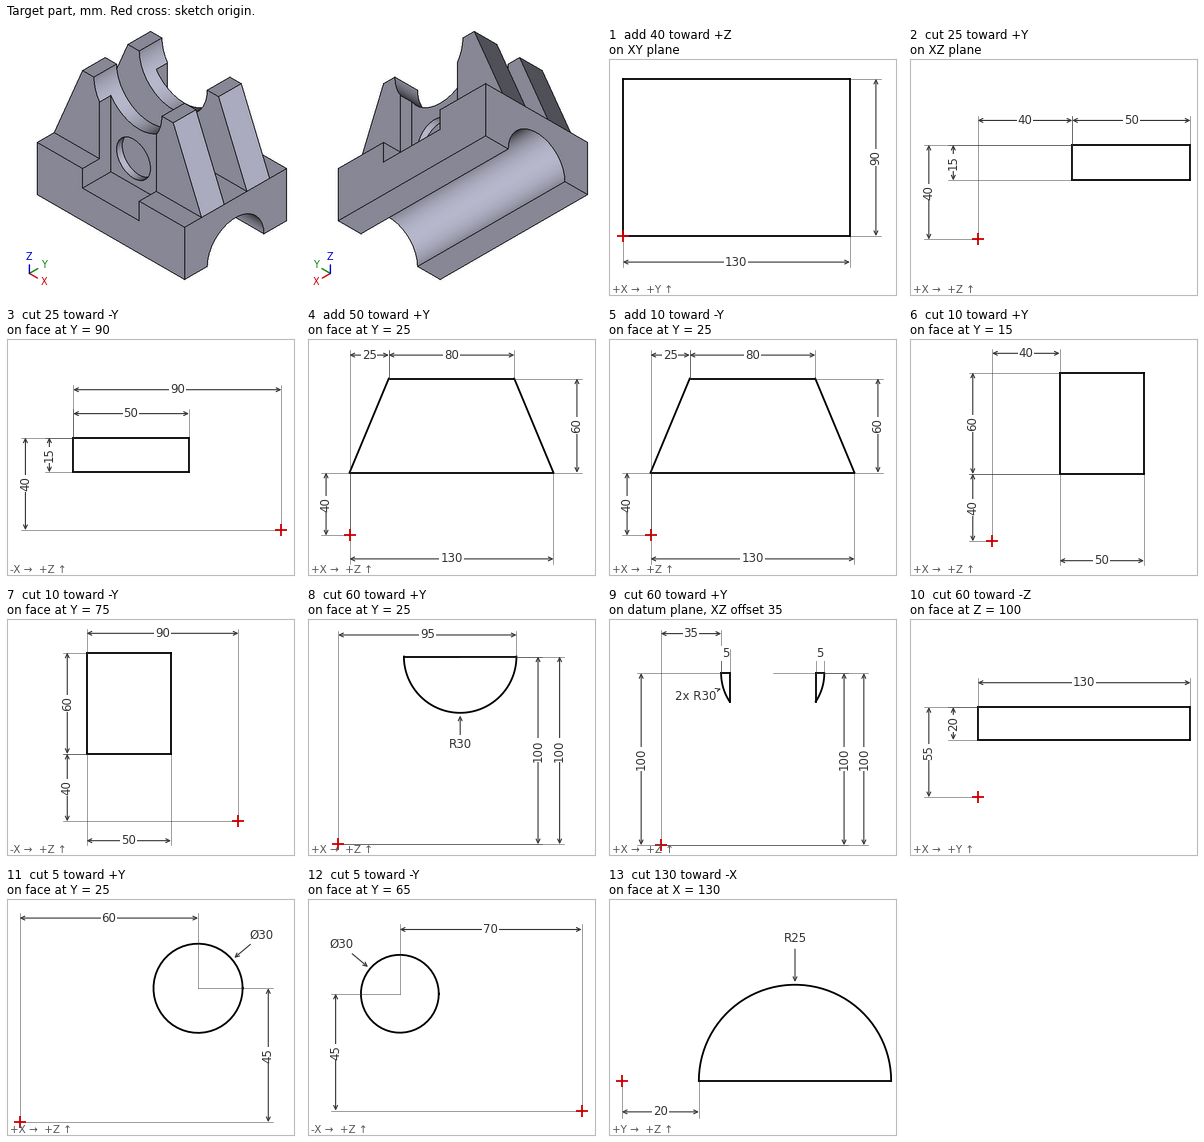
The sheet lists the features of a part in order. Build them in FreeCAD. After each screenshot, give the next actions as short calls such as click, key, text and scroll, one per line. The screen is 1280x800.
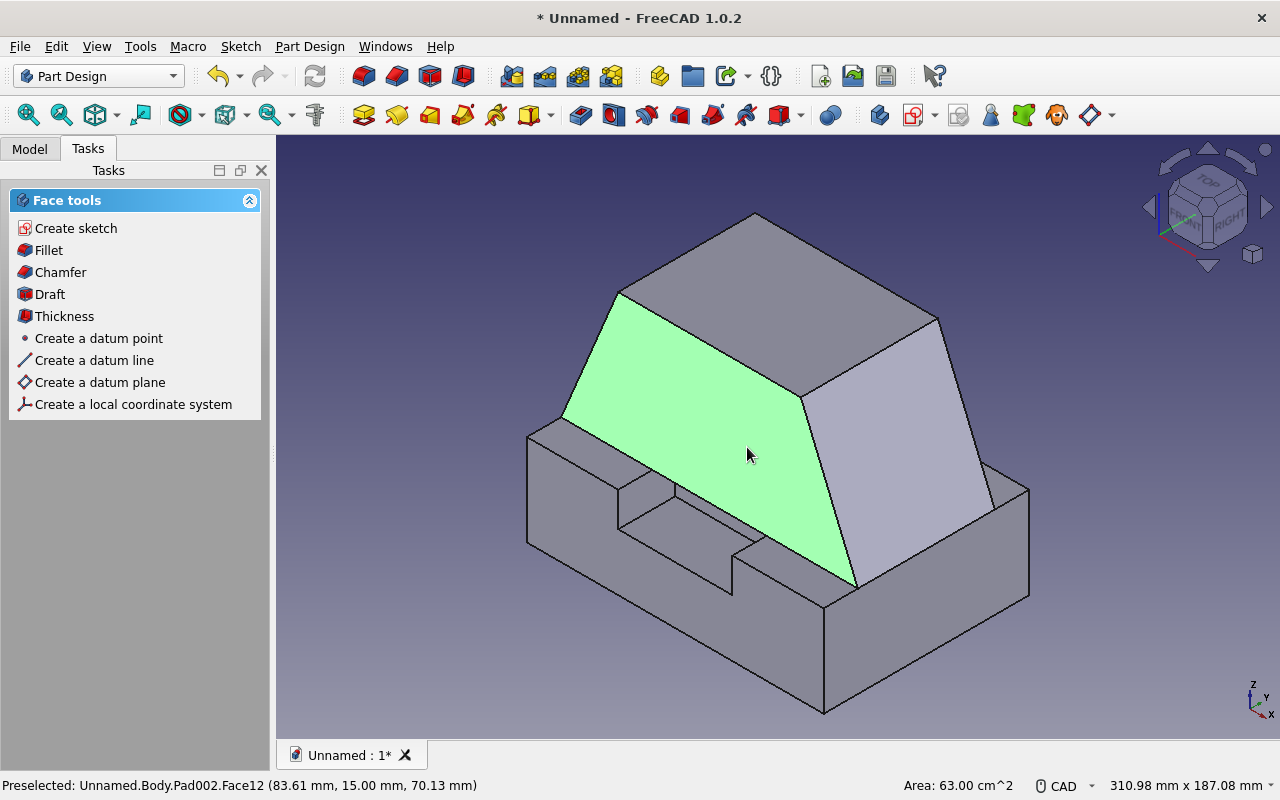
click(912, 116)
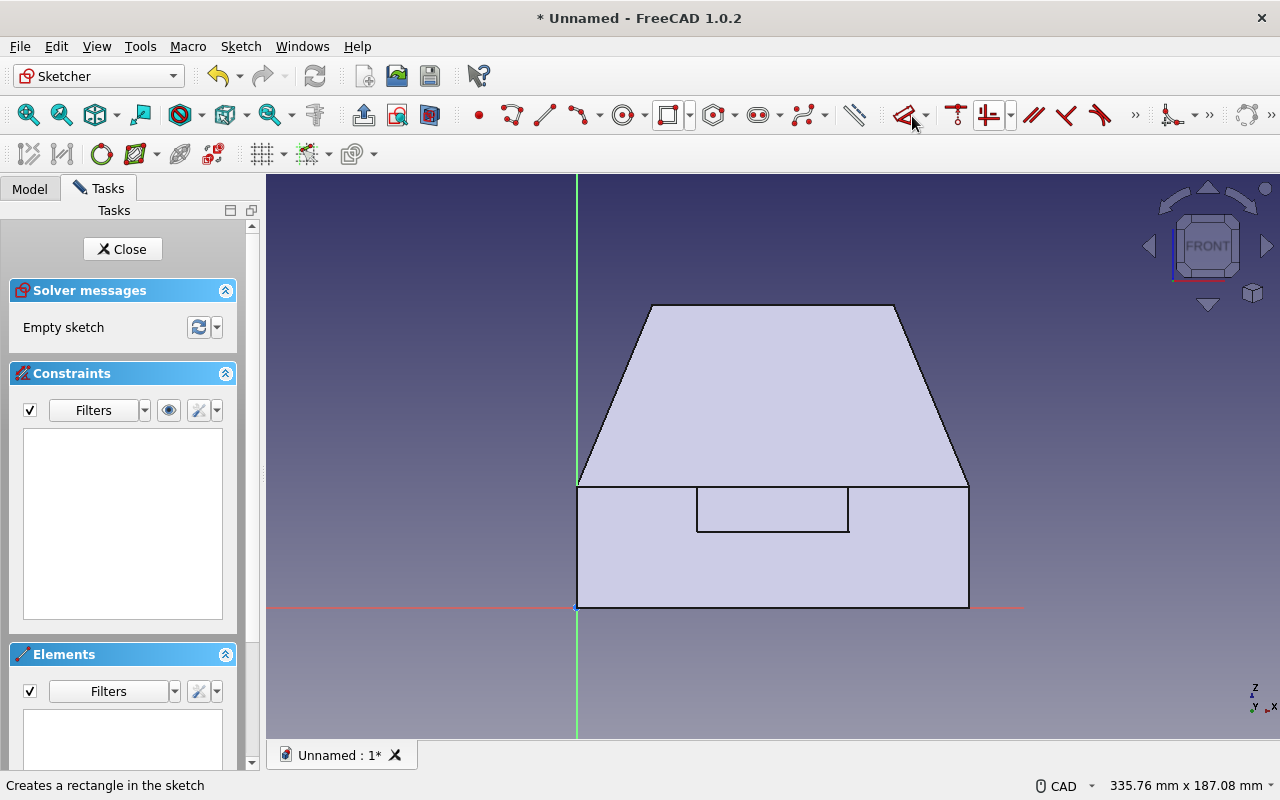
key(q)
key(s)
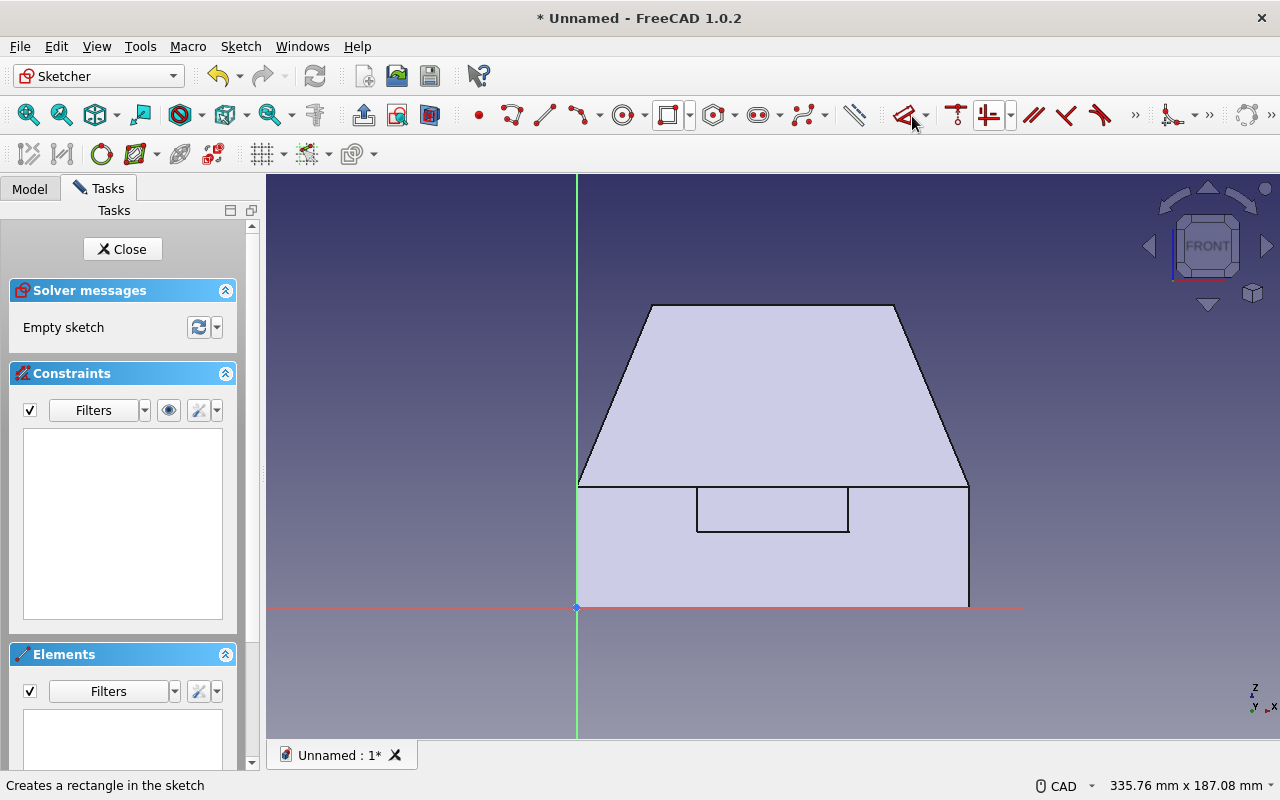
key(g)
key(r)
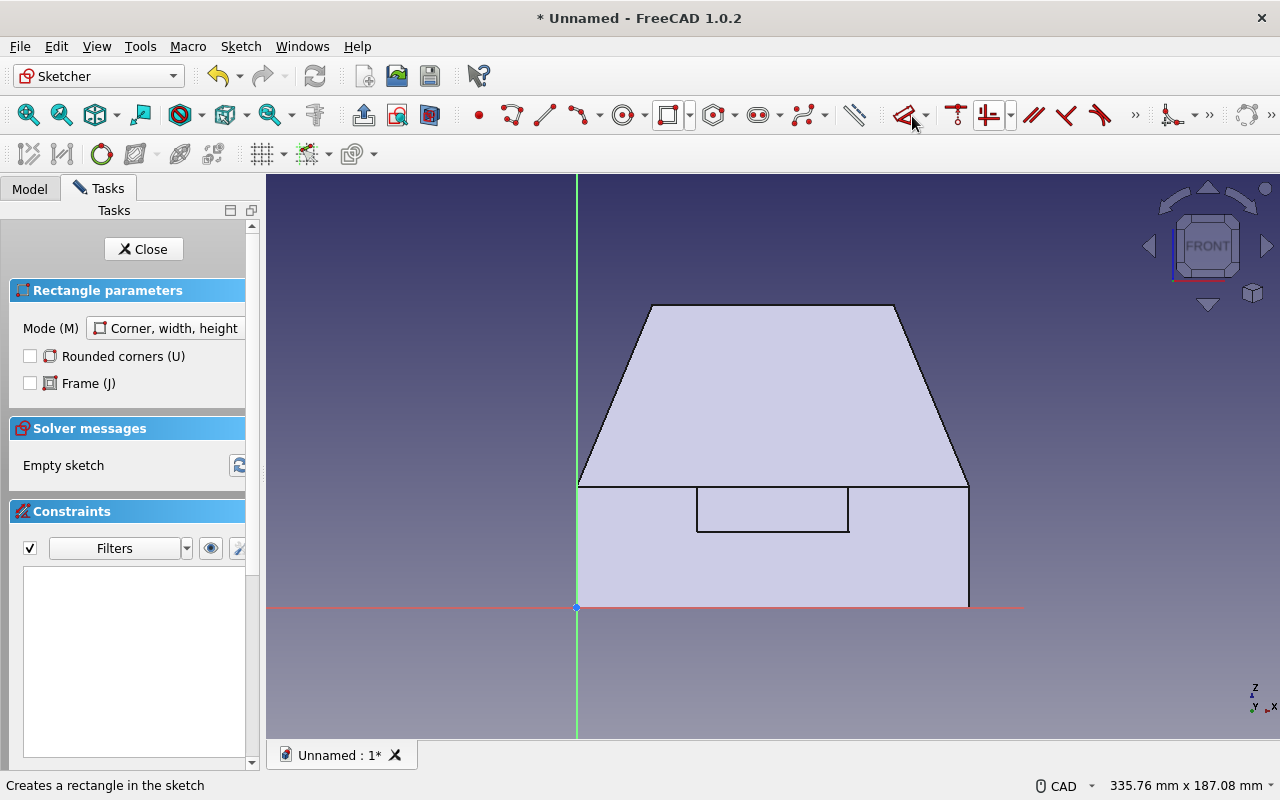
click(697, 305)
click(849, 487)
key(Escape)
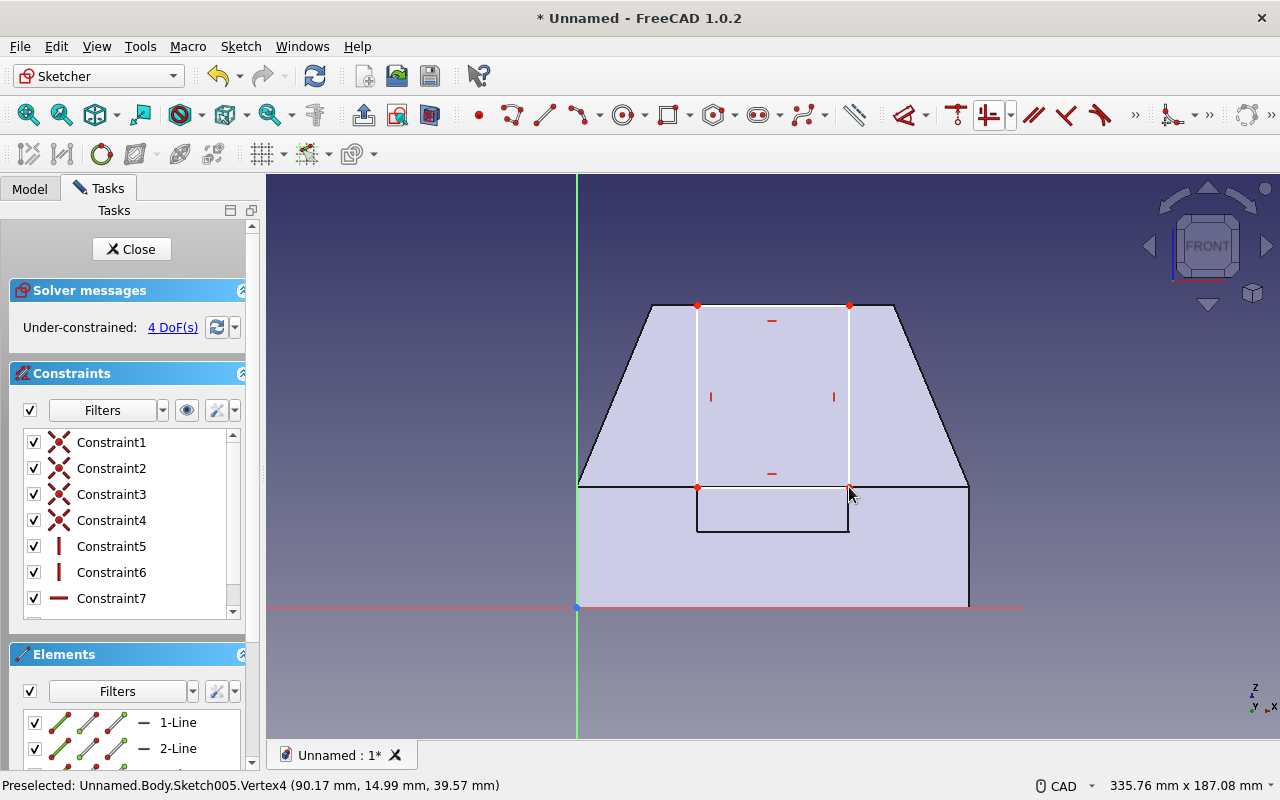
key(d)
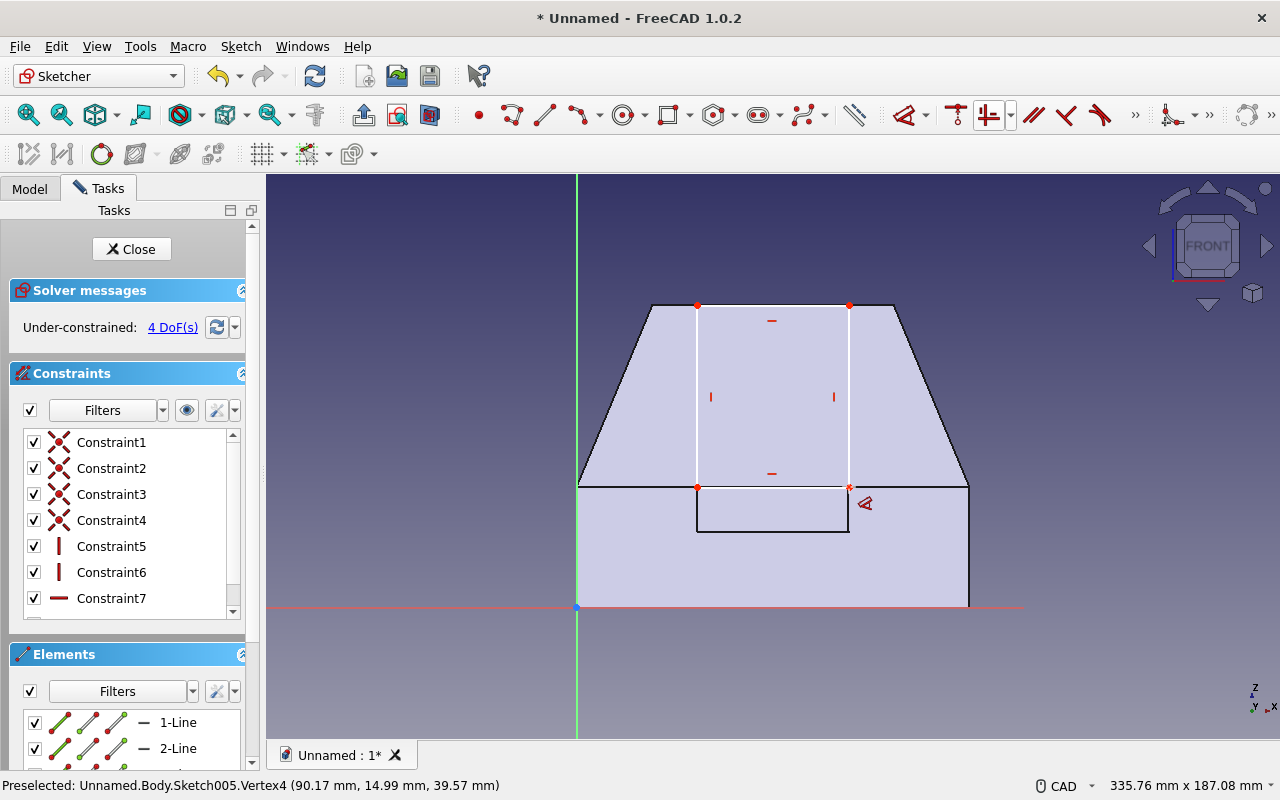
click(697, 361)
click(663, 397)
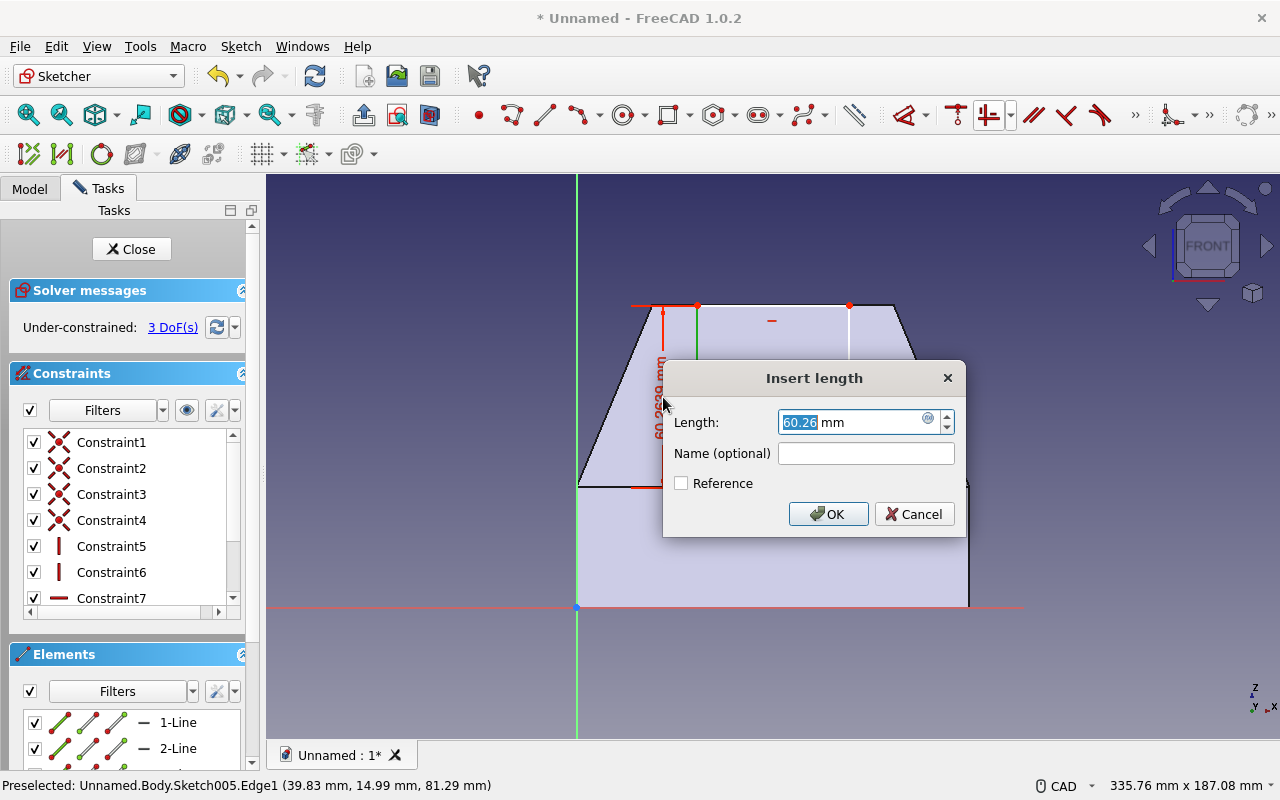
text(60)
key(Return)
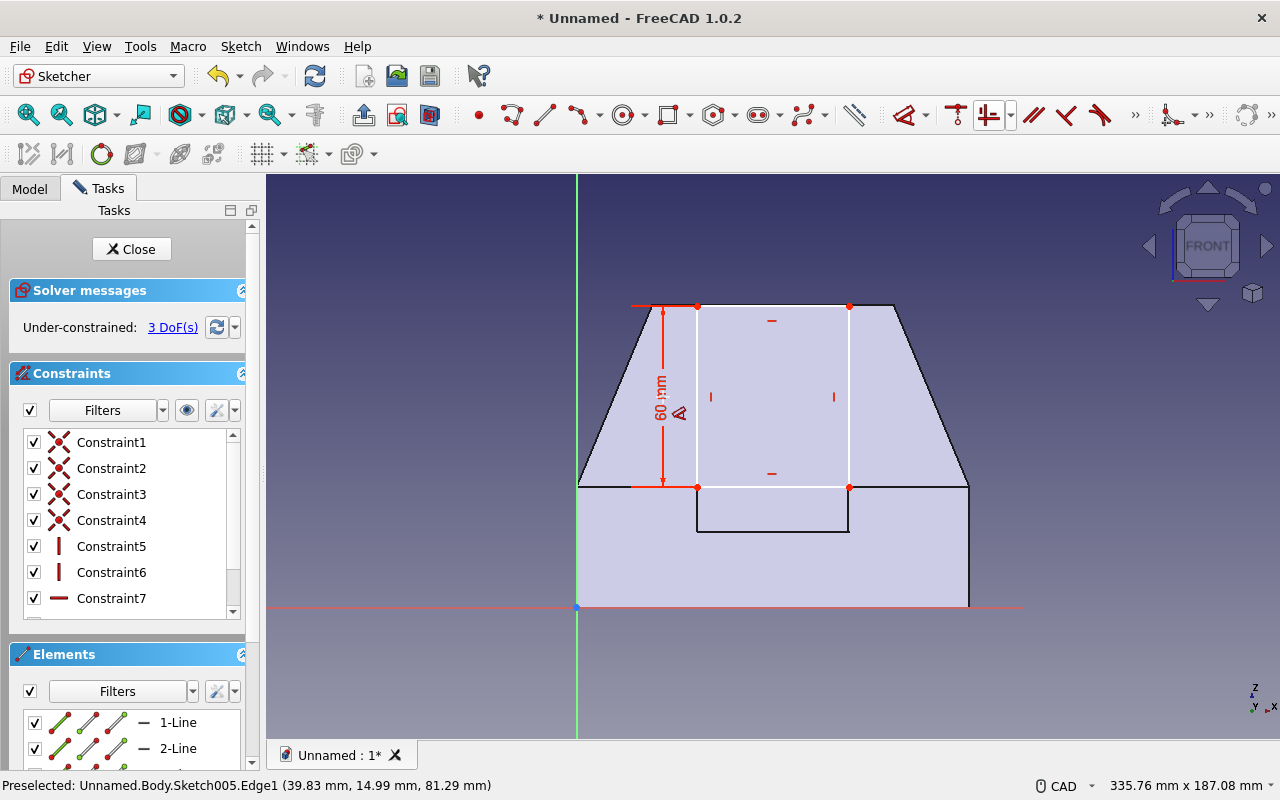
click(743, 487)
click(773, 521)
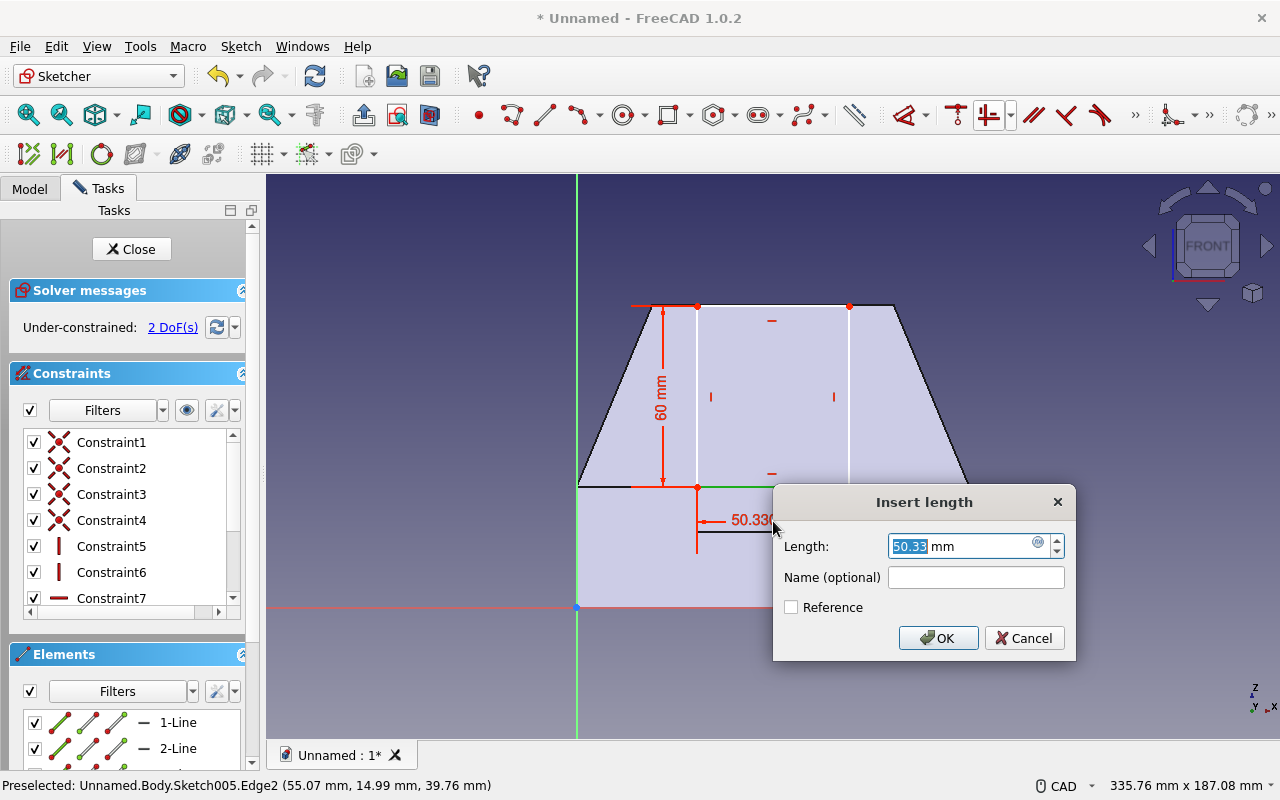
text(50)
key(Return)